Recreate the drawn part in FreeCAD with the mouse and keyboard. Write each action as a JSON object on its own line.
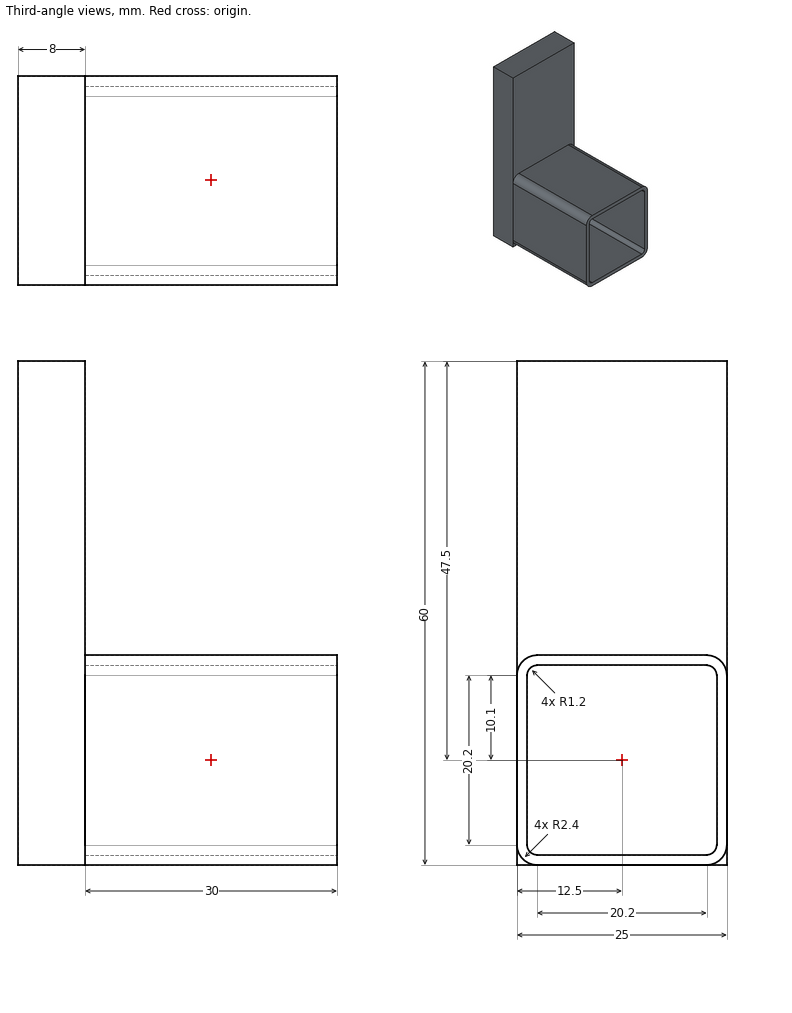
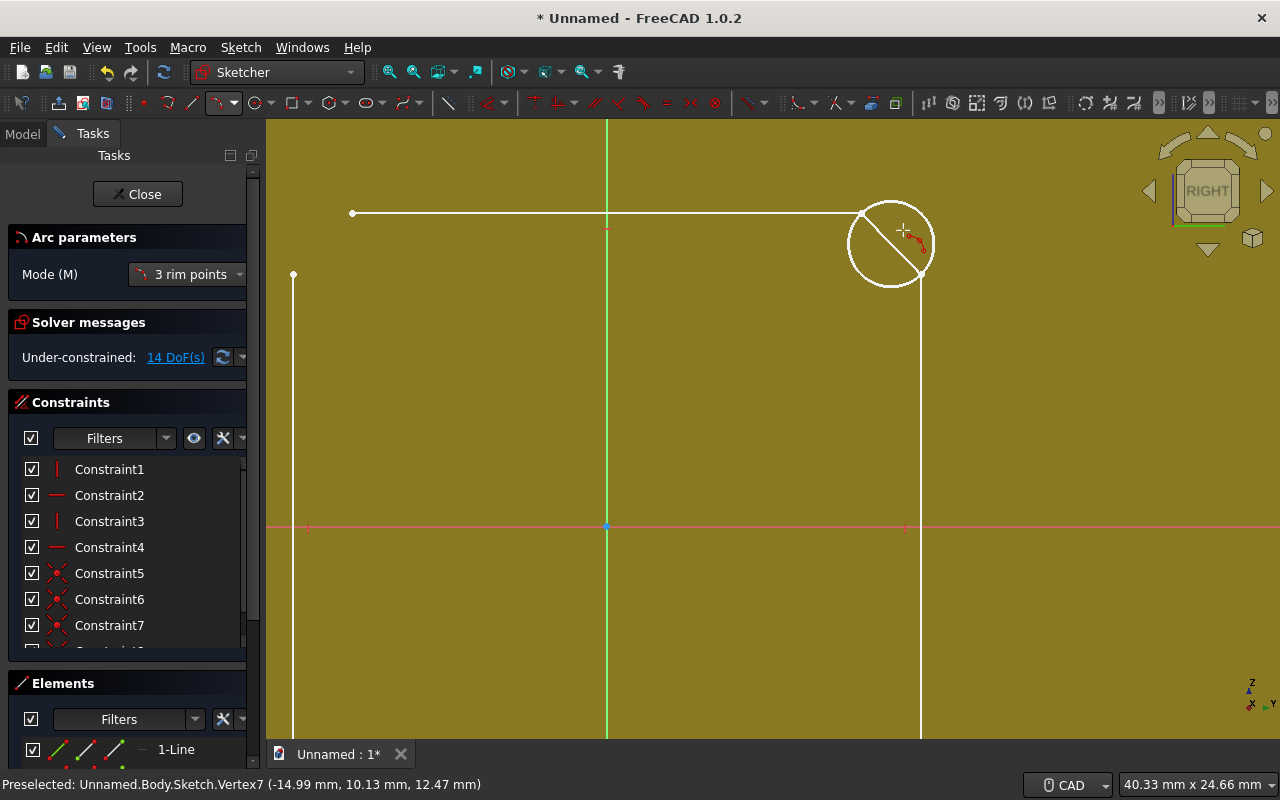
{"action": "left_click", "coordinate": [903, 230]}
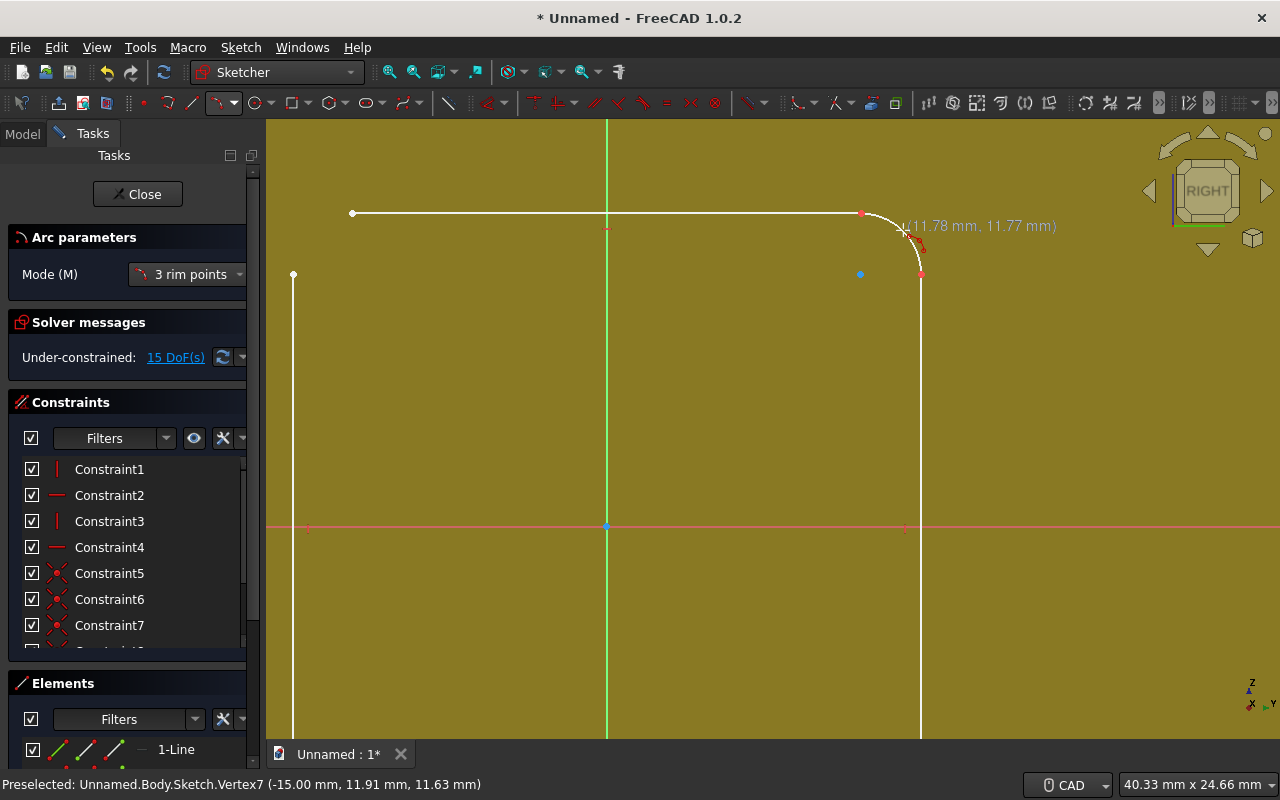
{"action": "left_click", "coordinate": [353, 213]}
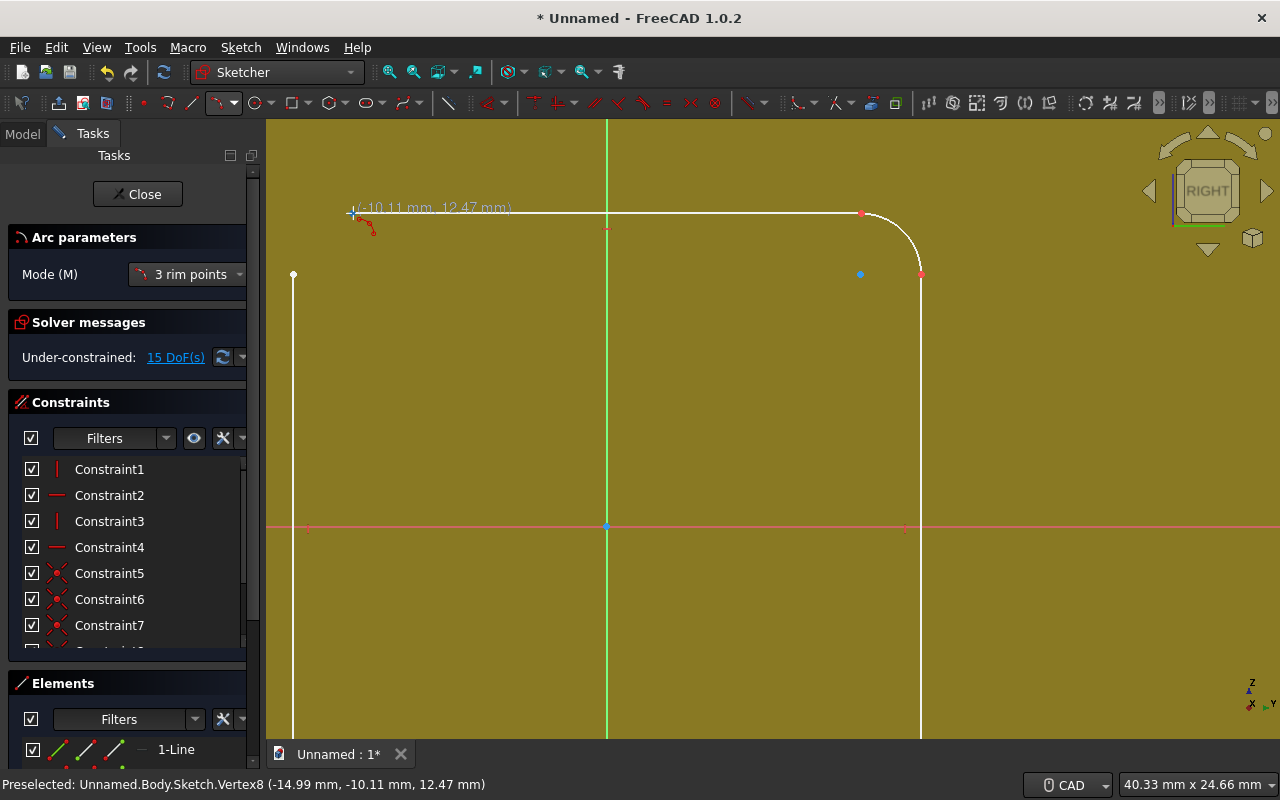
{"action": "scroll", "coordinate": [903, 230], "scroll_direction": "down", "scroll_amount": 2}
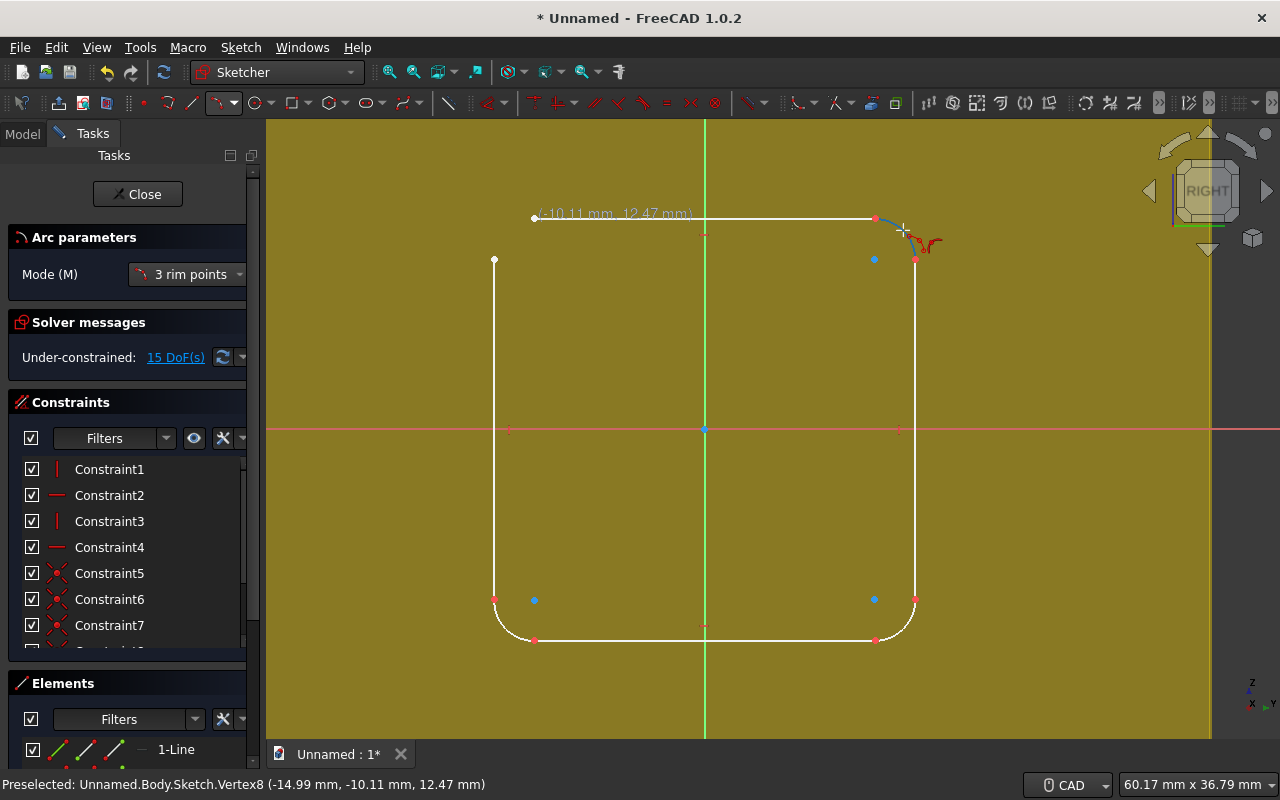
{"action": "left_click", "coordinate": [494, 260]}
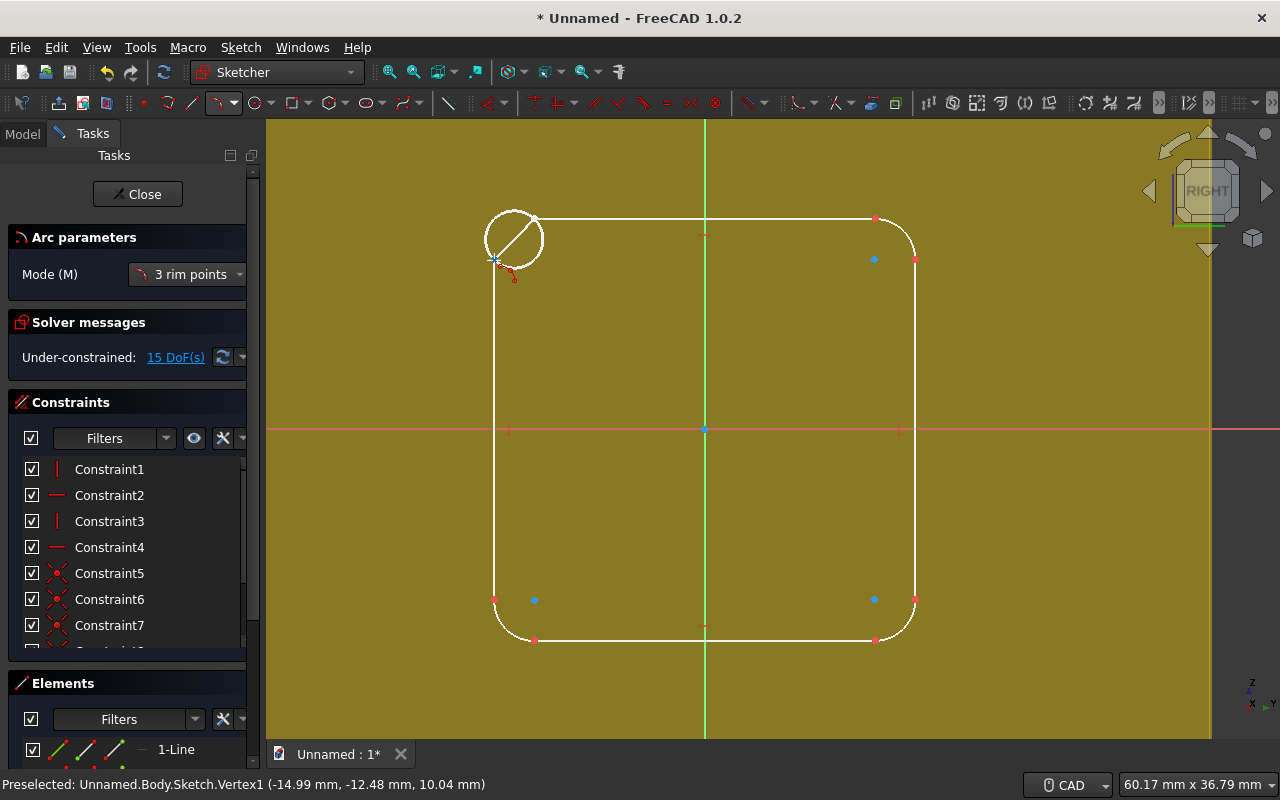
{"action": "scroll", "coordinate": [506, 230], "scroll_direction": "up", "scroll_amount": 2}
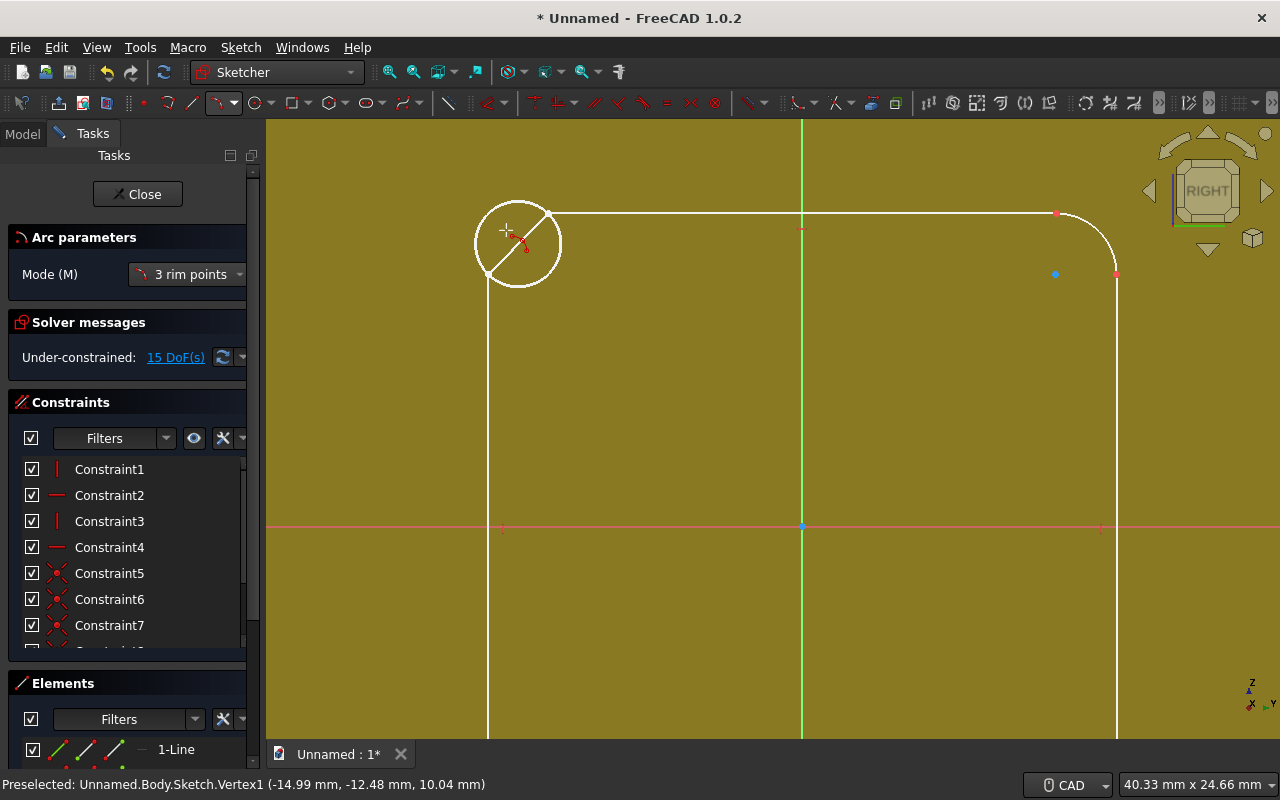
{"action": "left_click", "coordinate": [506, 230]}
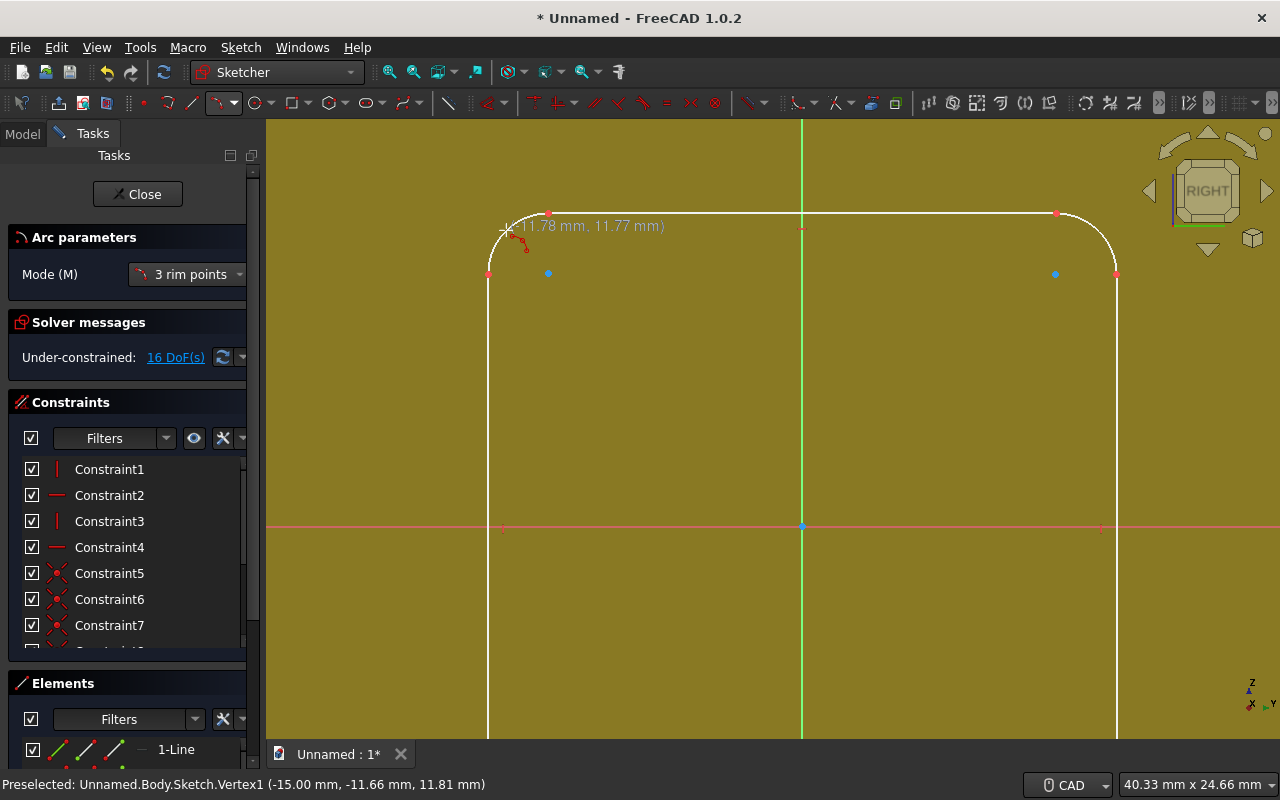
{"action": "key", "text": "g l"}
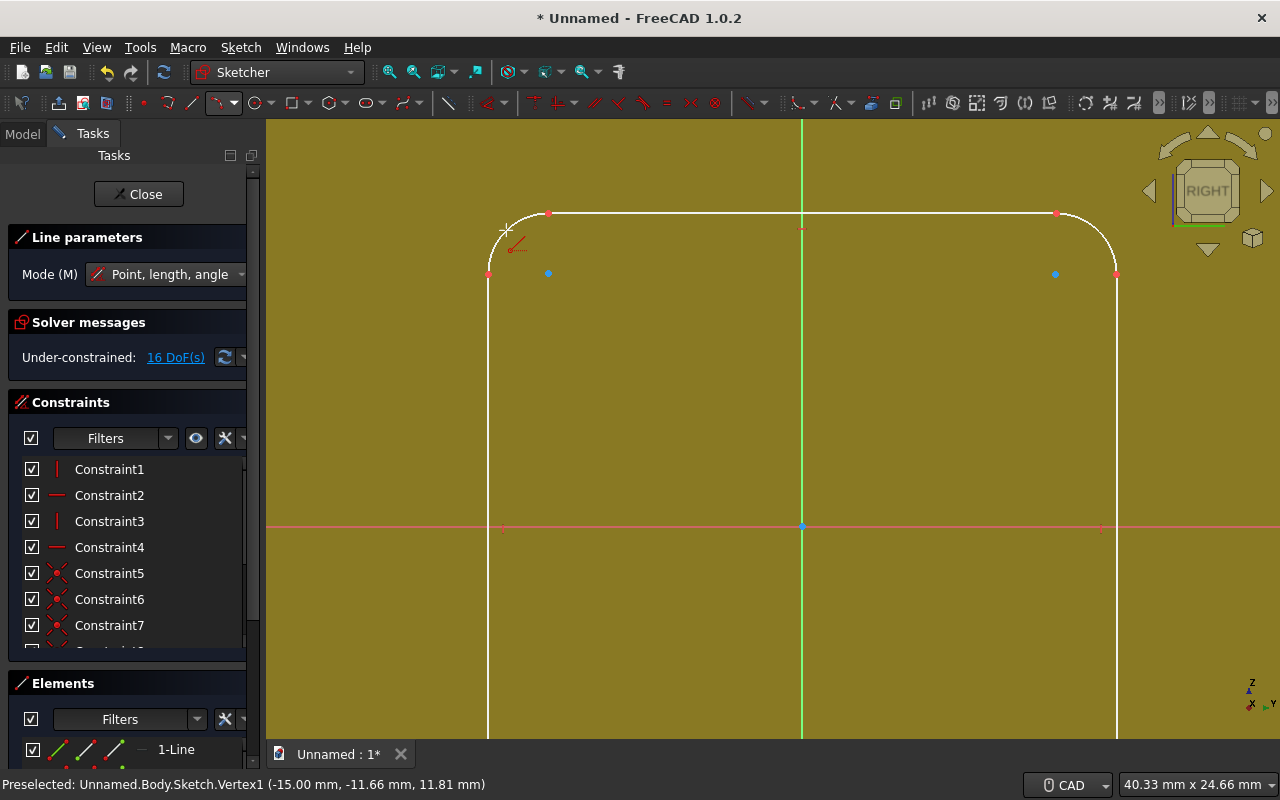
{"action": "scroll", "coordinate": [506, 230], "scroll_direction": "down", "scroll_amount": 2}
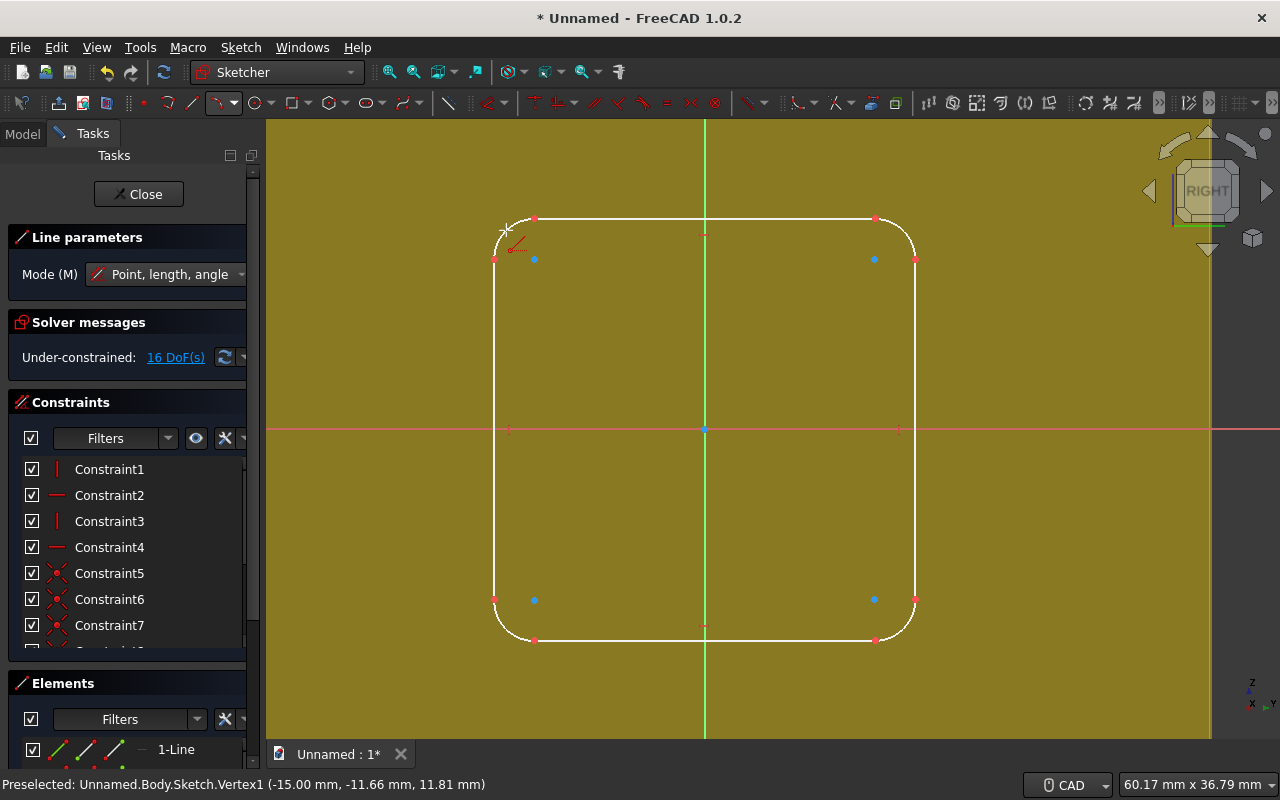
{"action": "left_click", "coordinate": [514, 599]}
{"action": "left_click", "coordinate": [514, 259]}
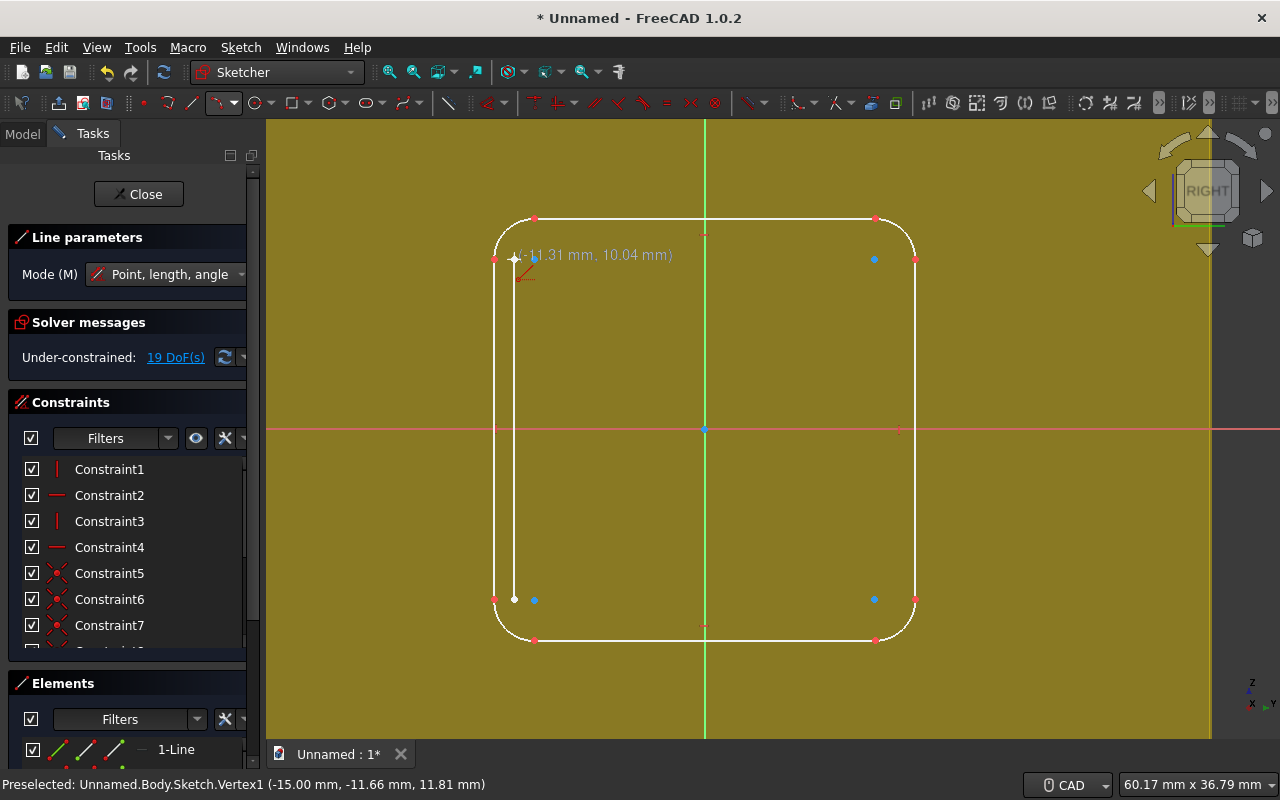
{"action": "left_click", "coordinate": [534, 239]}
{"action": "left_click", "coordinate": [875, 239]}